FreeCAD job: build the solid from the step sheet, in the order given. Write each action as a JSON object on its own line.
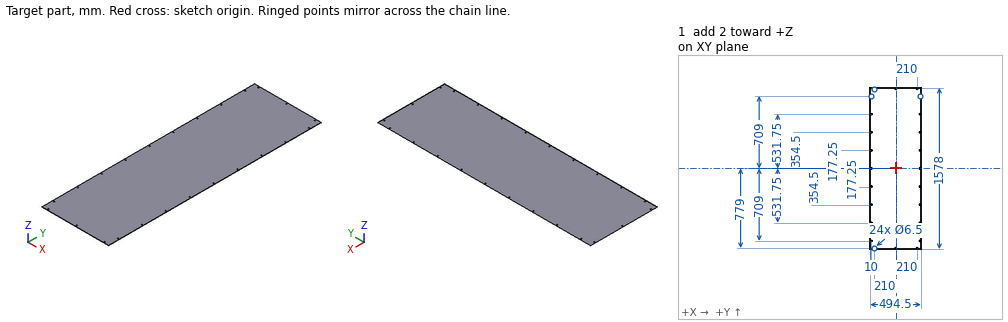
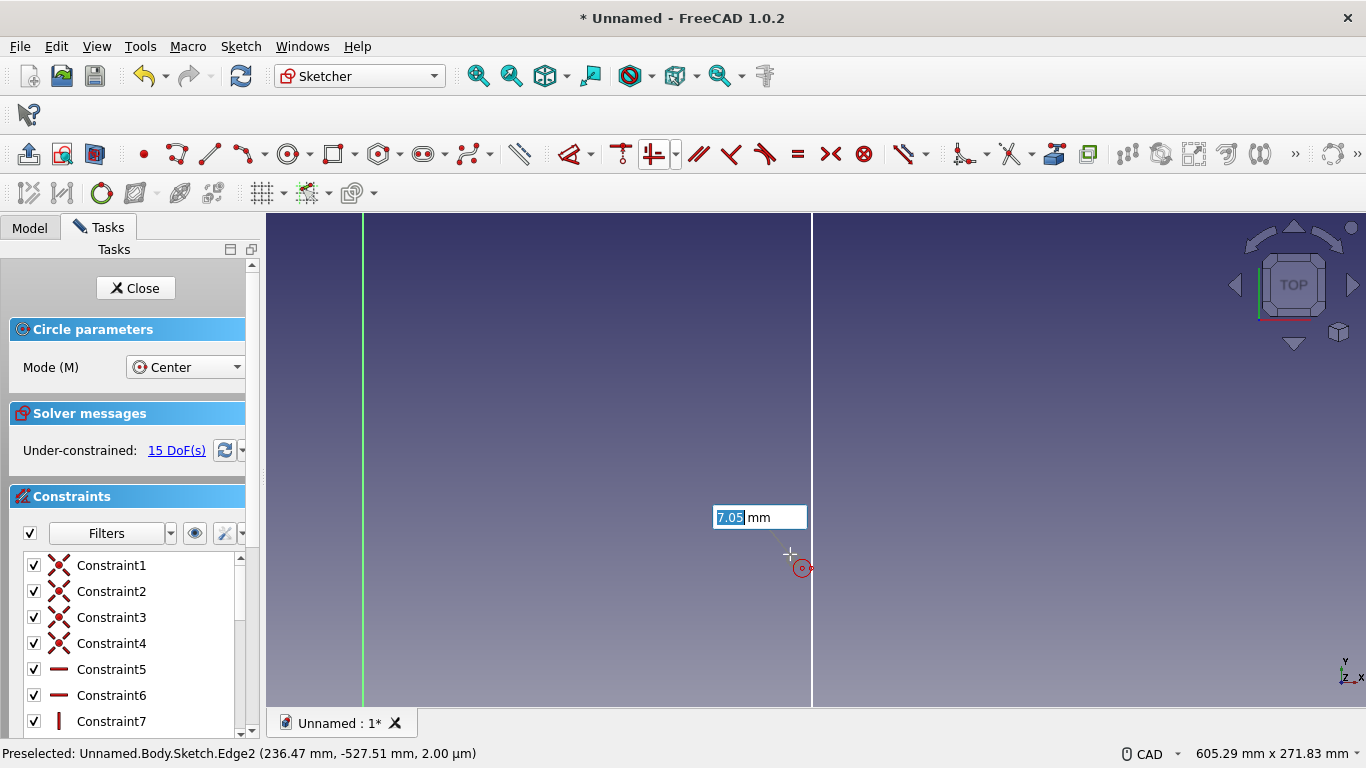
{"action": "type", "text": "6.5"}
{"action": "key", "text": "Return"}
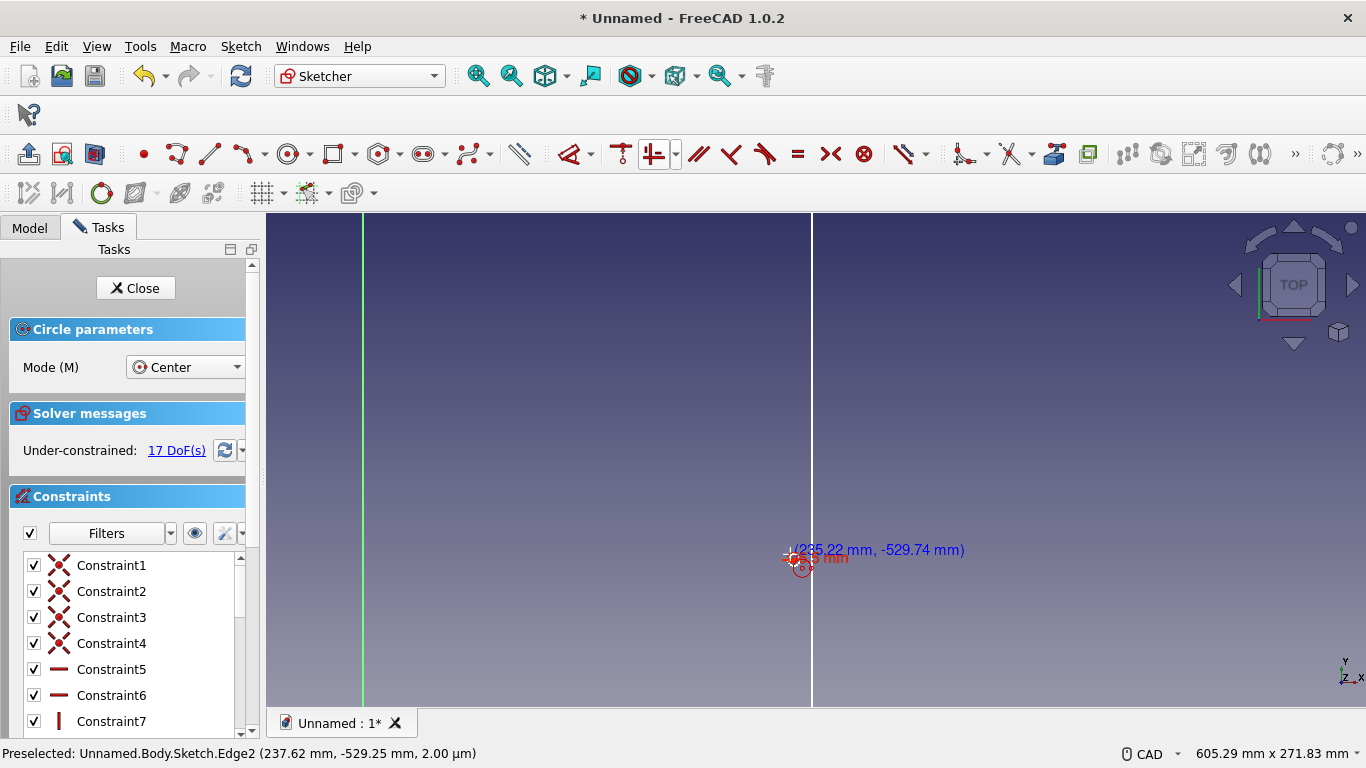
{"action": "scroll", "coordinate": [795, 568], "scroll_direction": "down", "scroll_amount": 11}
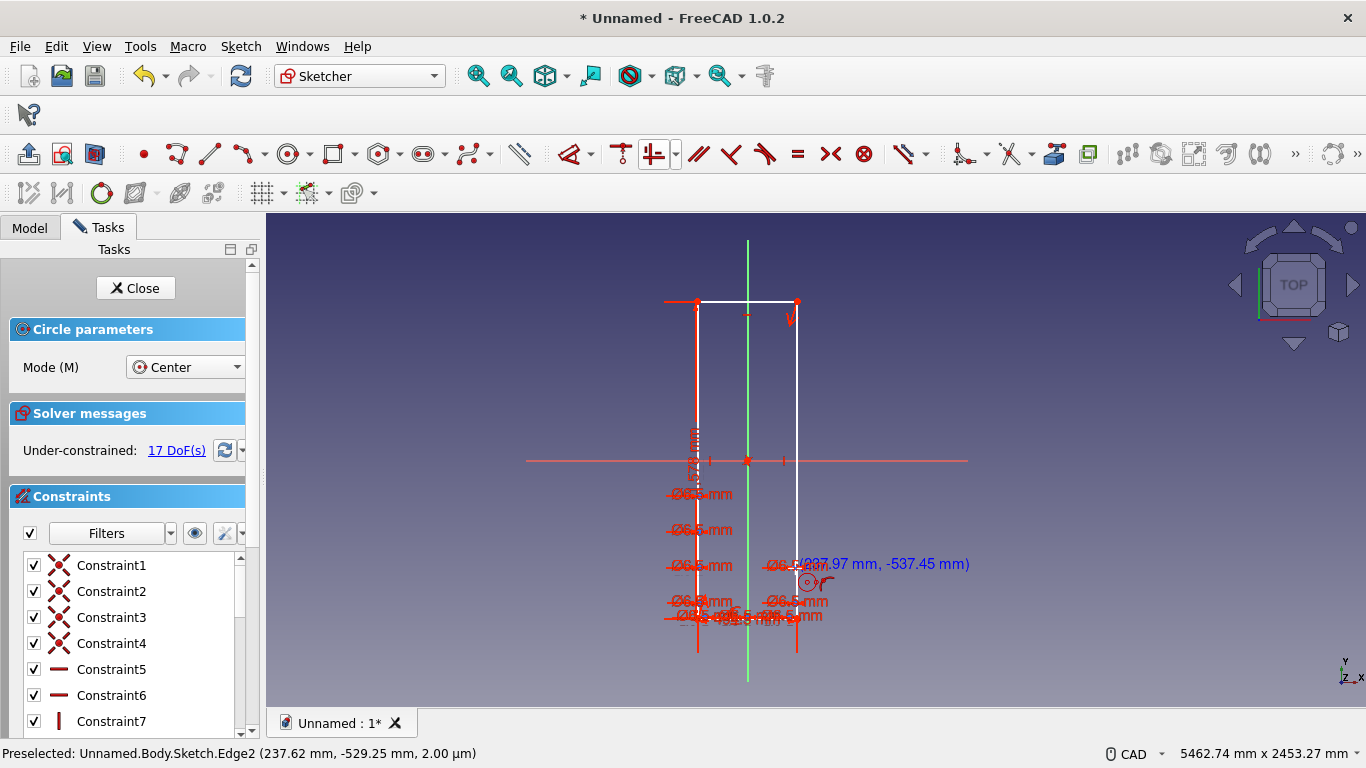
{"action": "scroll", "coordinate": [795, 532], "scroll_direction": "up", "scroll_amount": 18}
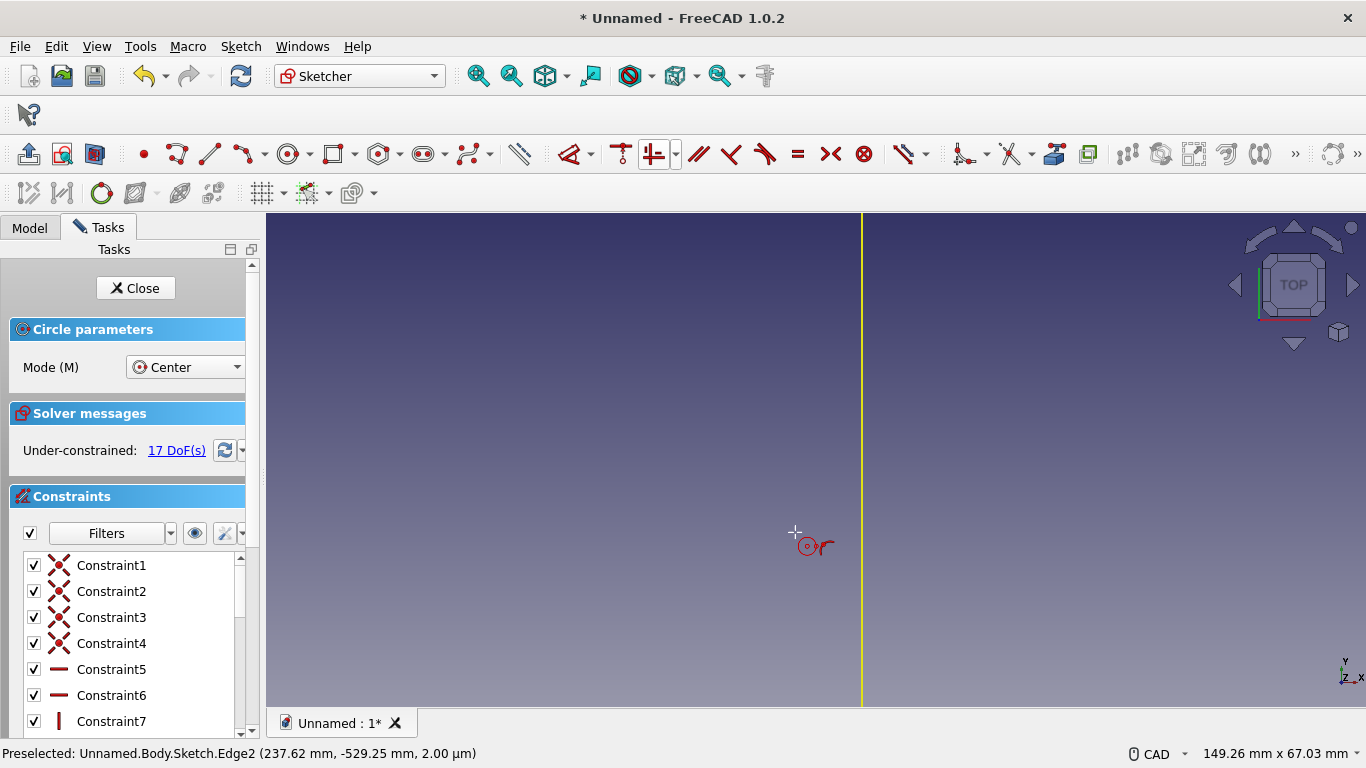
{"action": "scroll", "coordinate": [795, 532], "scroll_direction": "down", "scroll_amount": 18}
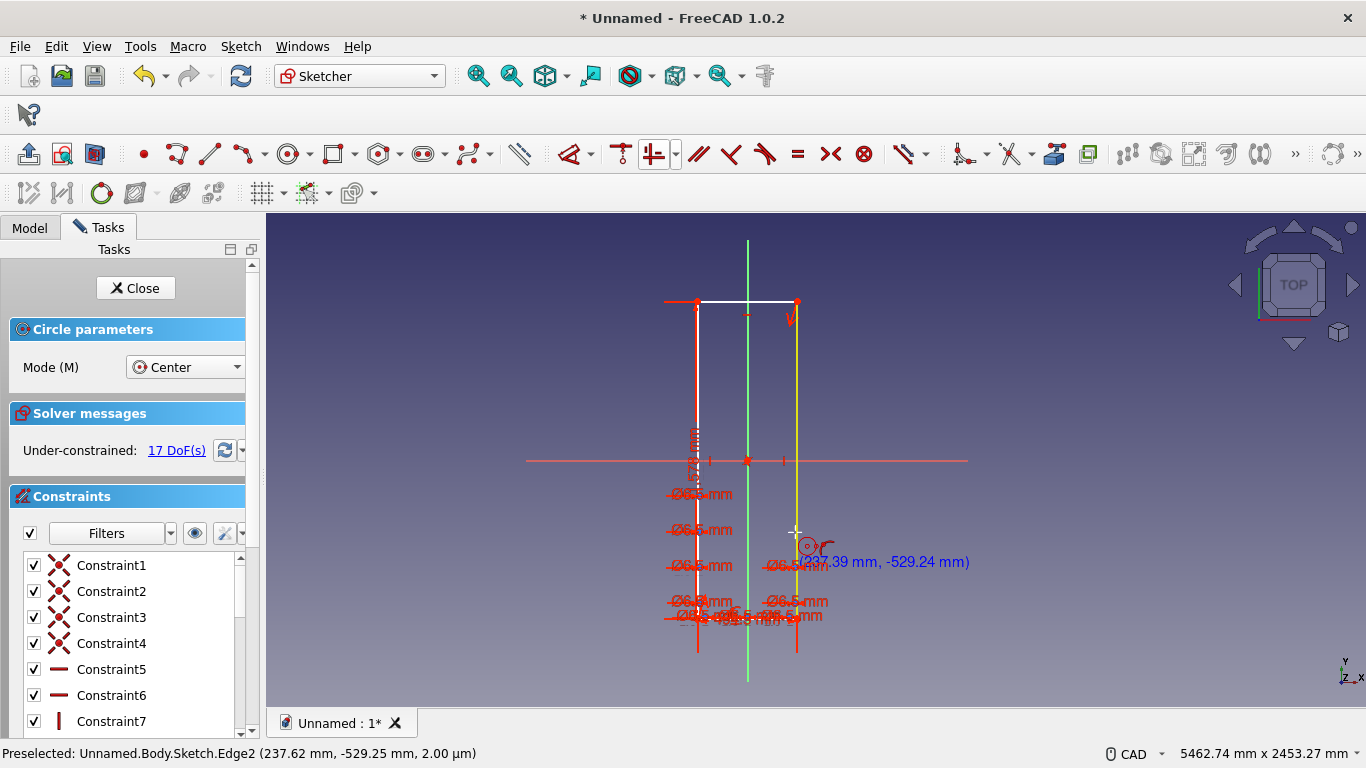
{"action": "scroll", "coordinate": [795, 532], "scroll_direction": "up", "scroll_amount": 11}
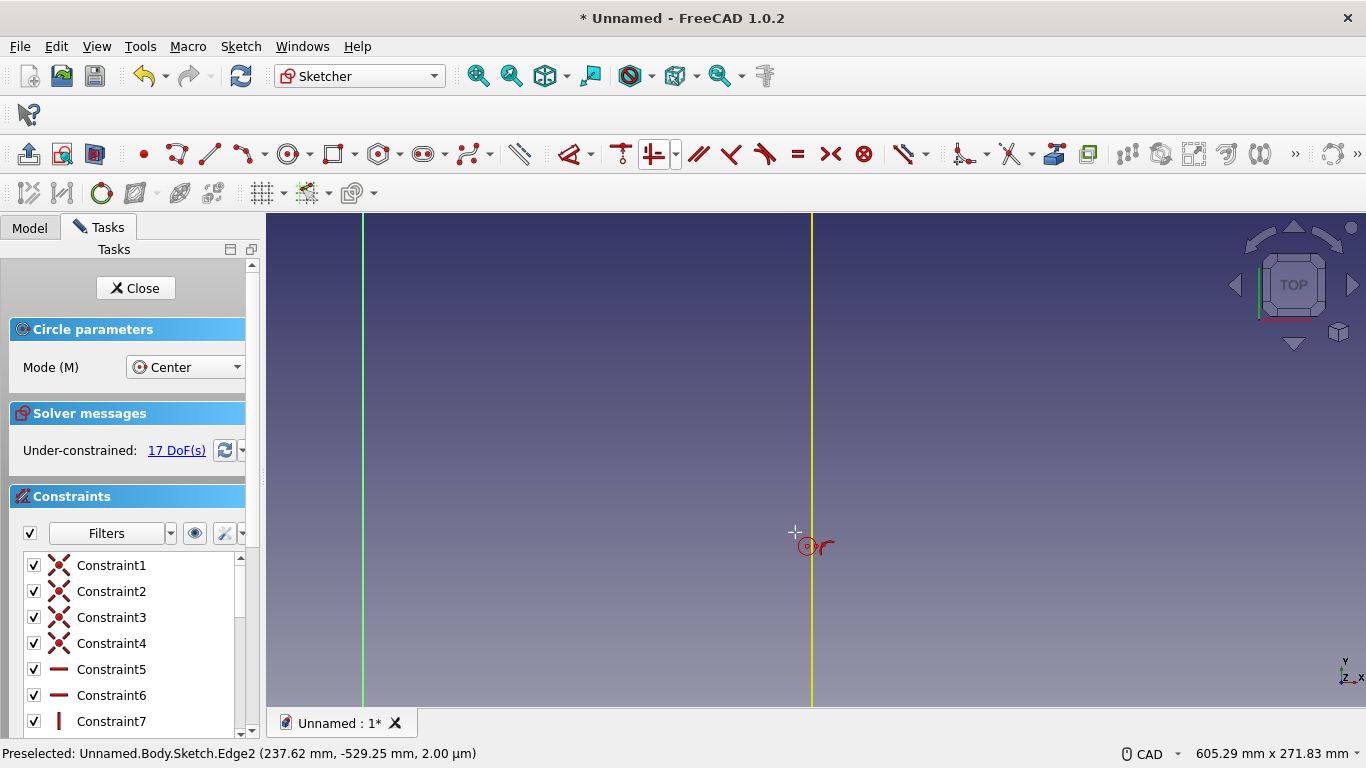
{"action": "left_click", "coordinate": [794, 526]}
{"action": "mouse_move", "coordinate": [790, 522]}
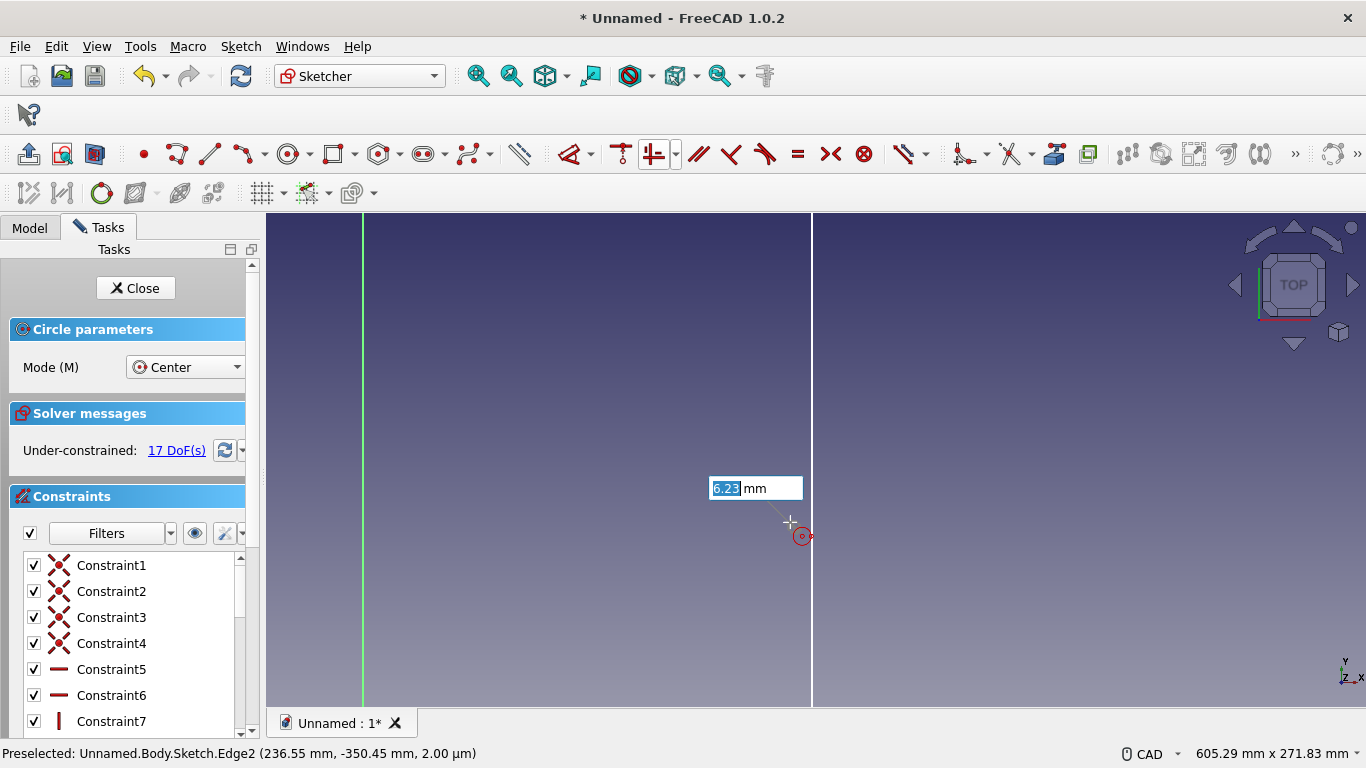
{"action": "type", "text": "6.5"}
{"action": "key", "text": "Return"}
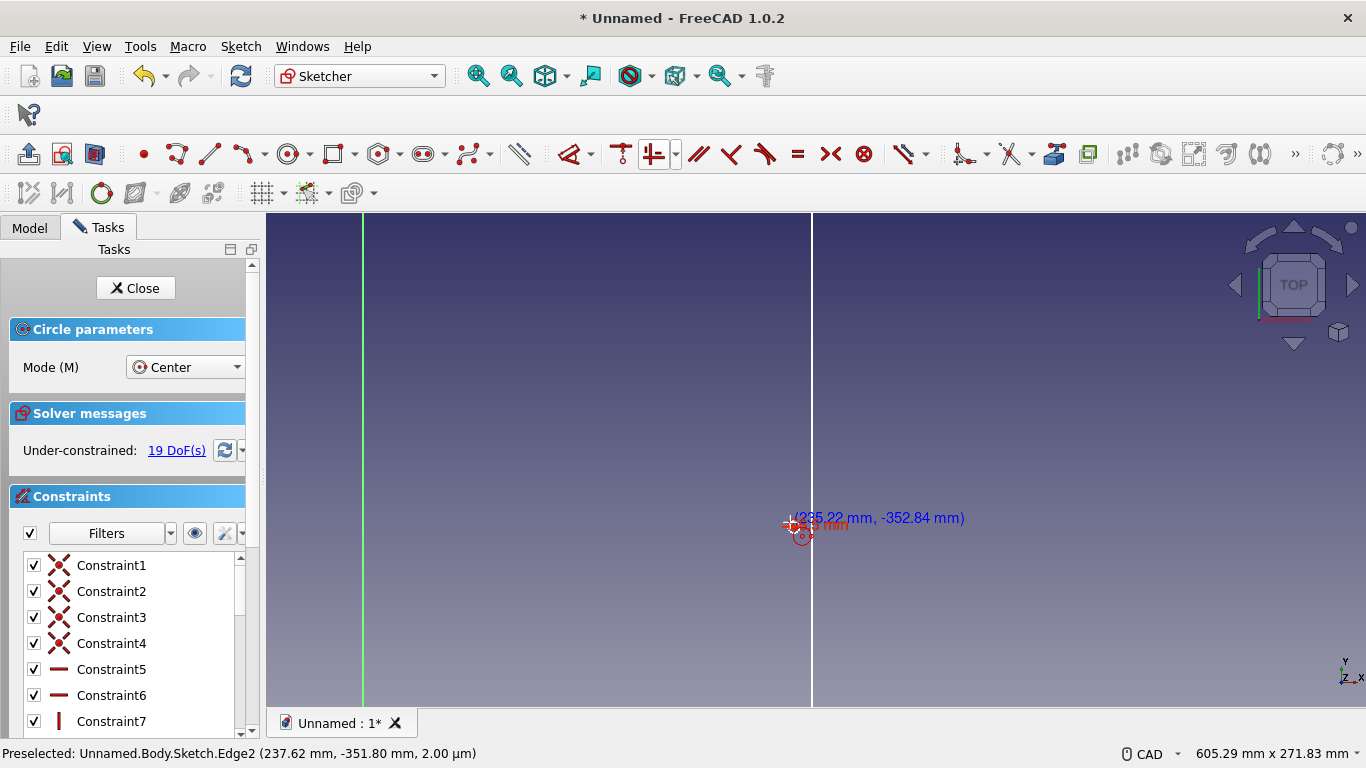
{"action": "scroll", "coordinate": [795, 532], "scroll_direction": "down", "scroll_amount": 11}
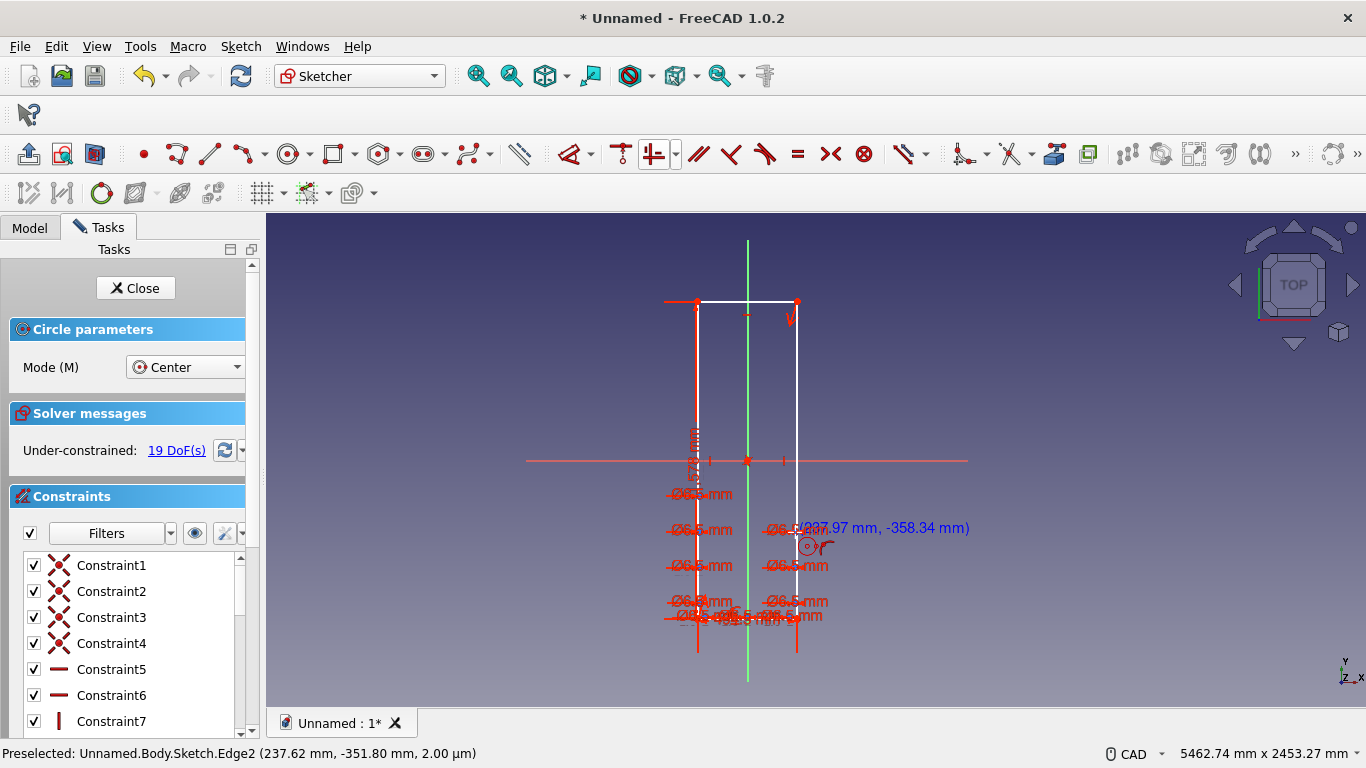
{"action": "scroll", "coordinate": [795, 496], "scroll_direction": "up", "scroll_amount": 18}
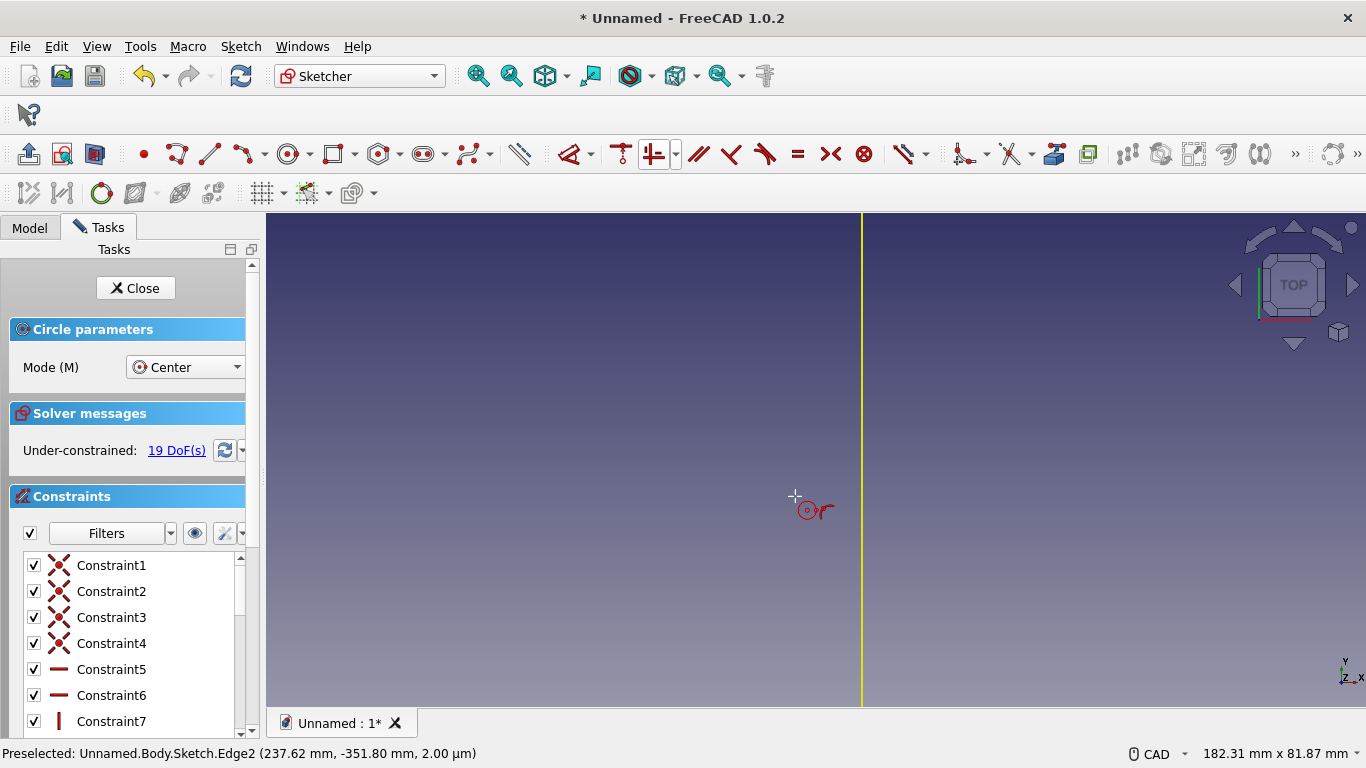
{"action": "scroll", "coordinate": [795, 496], "scroll_direction": "down", "scroll_amount": 18}